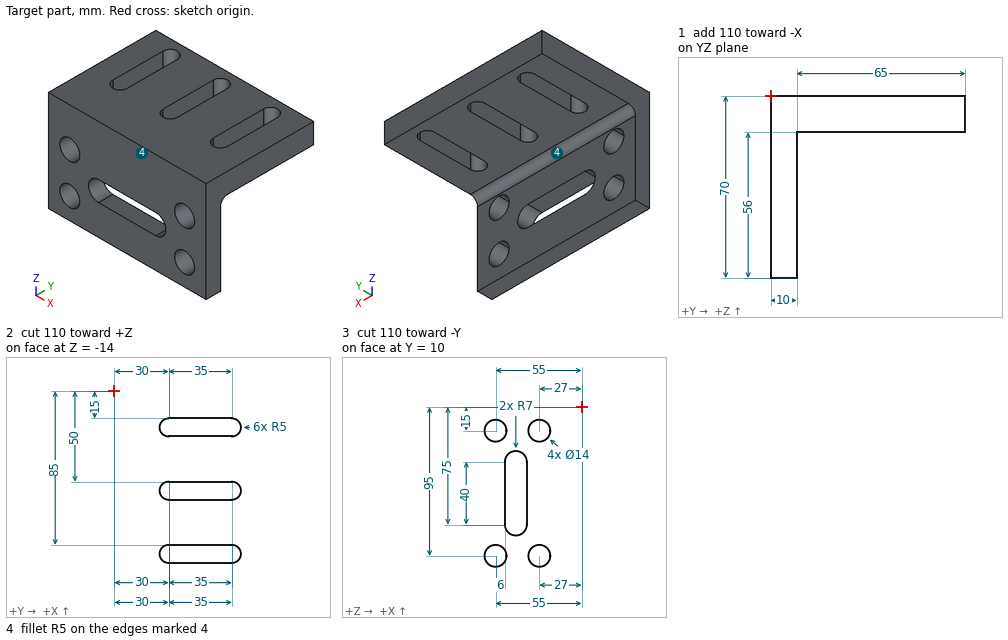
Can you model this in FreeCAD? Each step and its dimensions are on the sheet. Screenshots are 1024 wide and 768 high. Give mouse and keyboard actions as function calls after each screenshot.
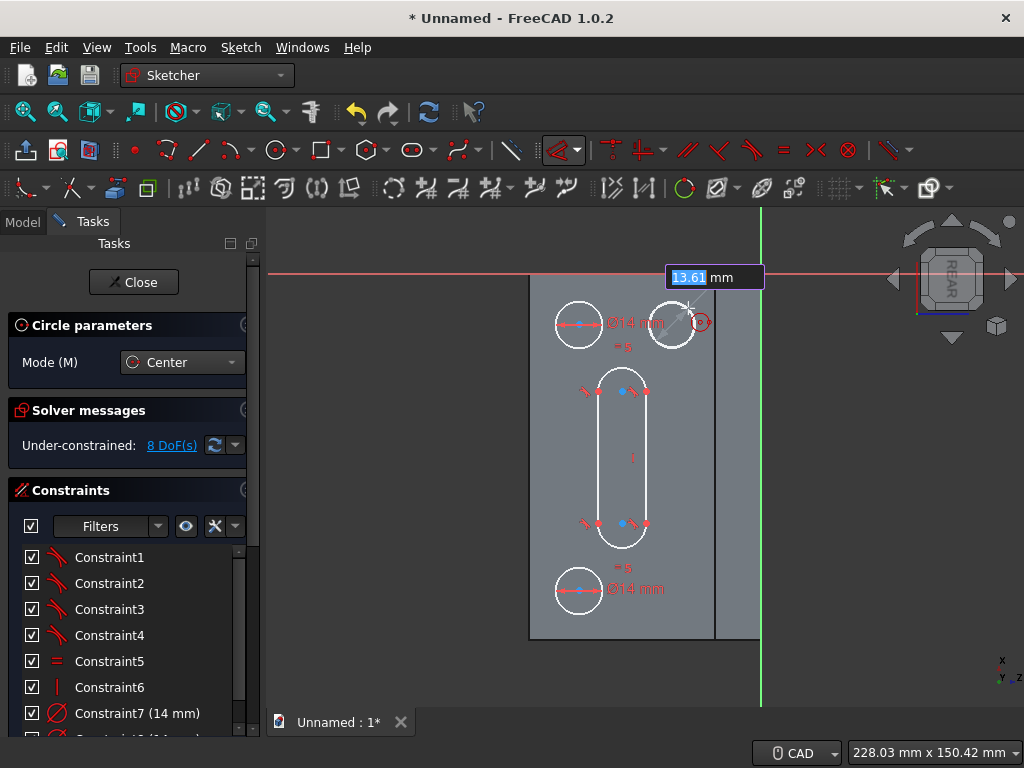
text(14)
key(Return)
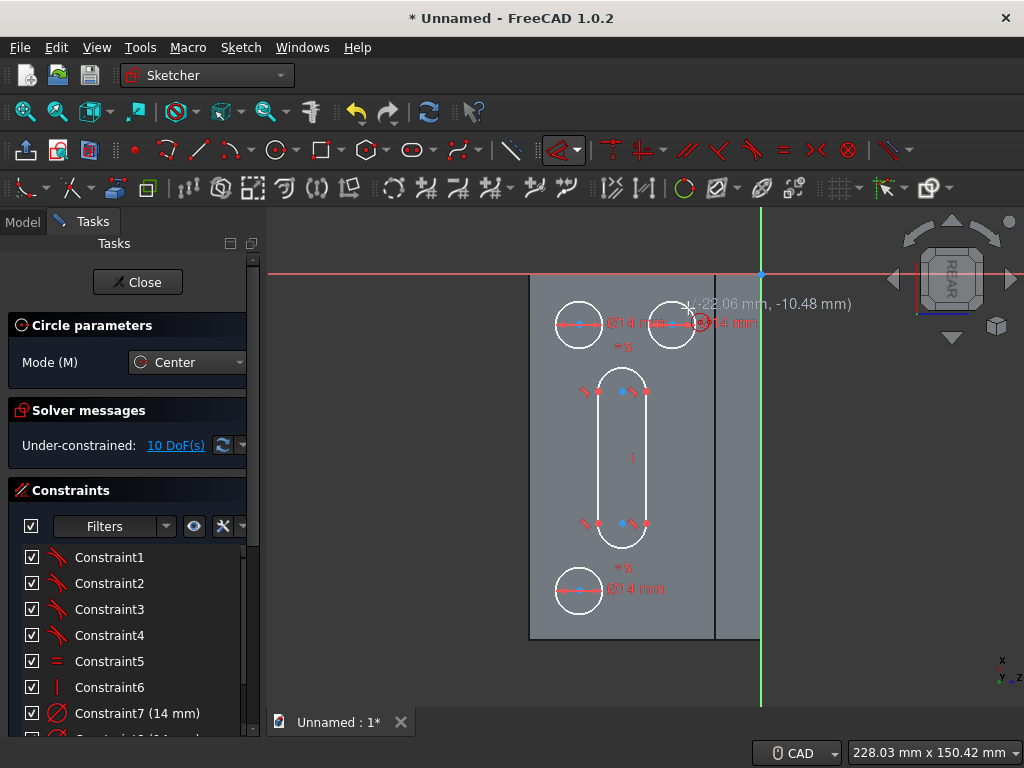
click(672, 590)
move(688, 574)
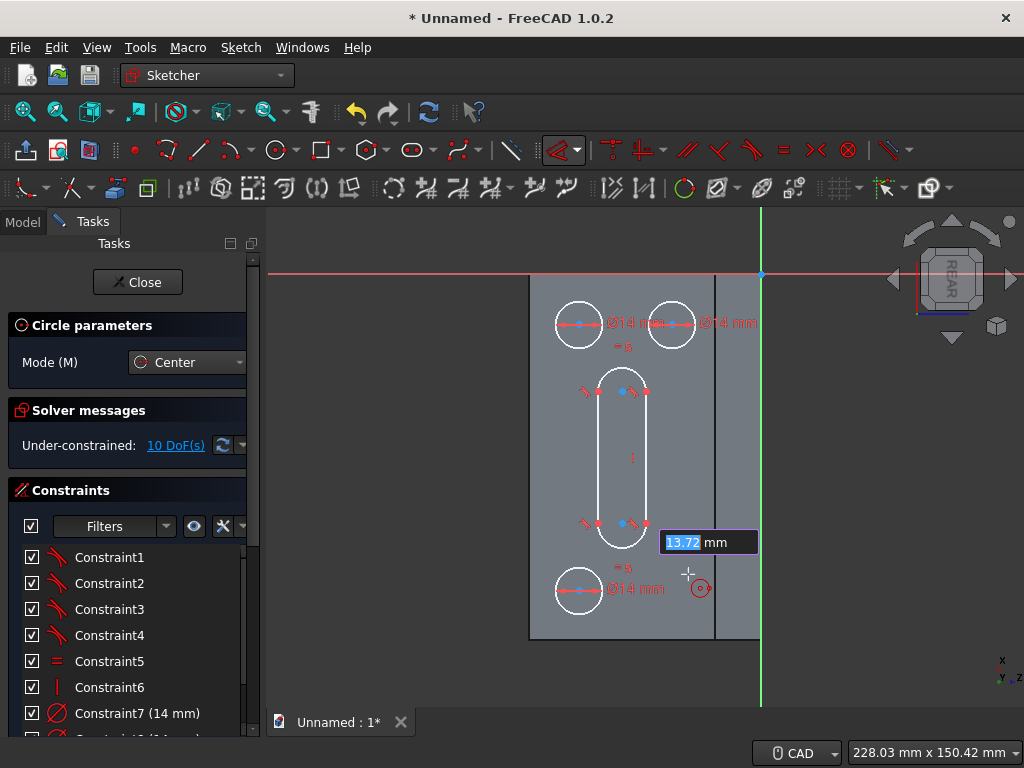
text(14)
key(Return)
key(Escape)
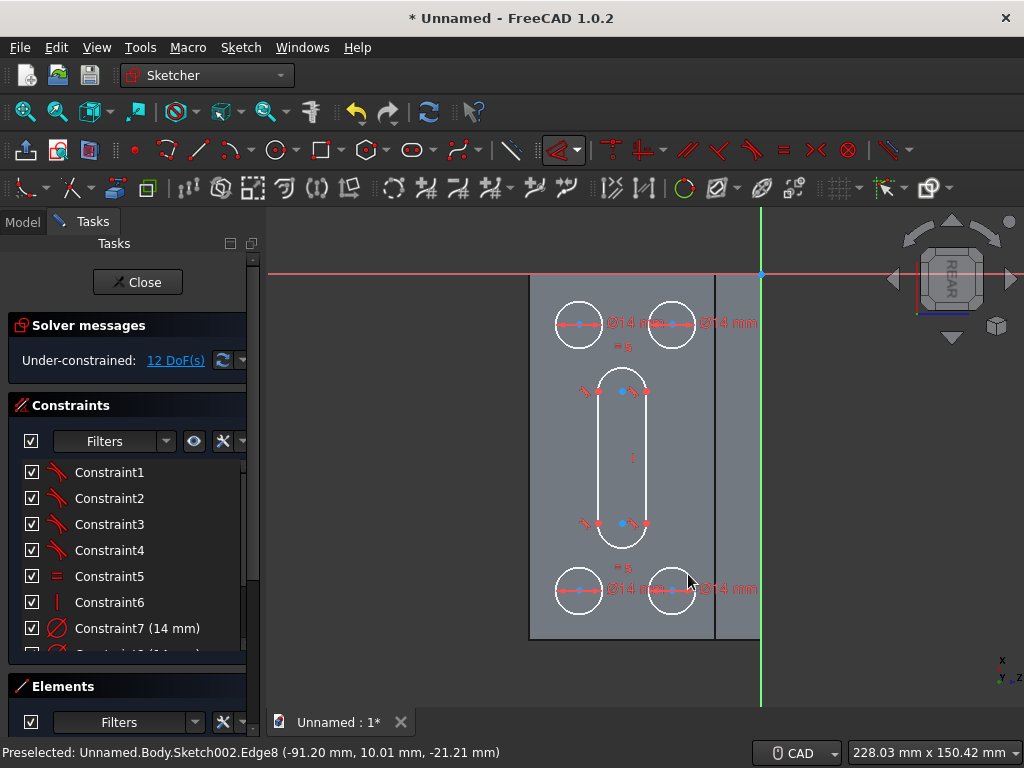
click(579, 325)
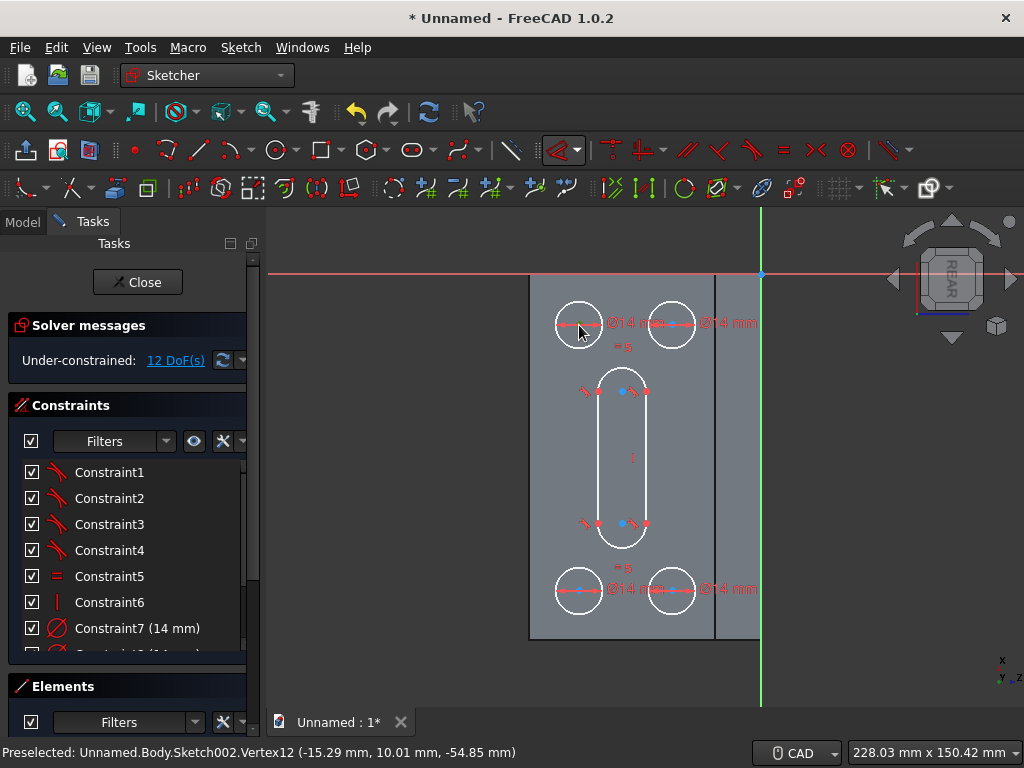
click(672, 325)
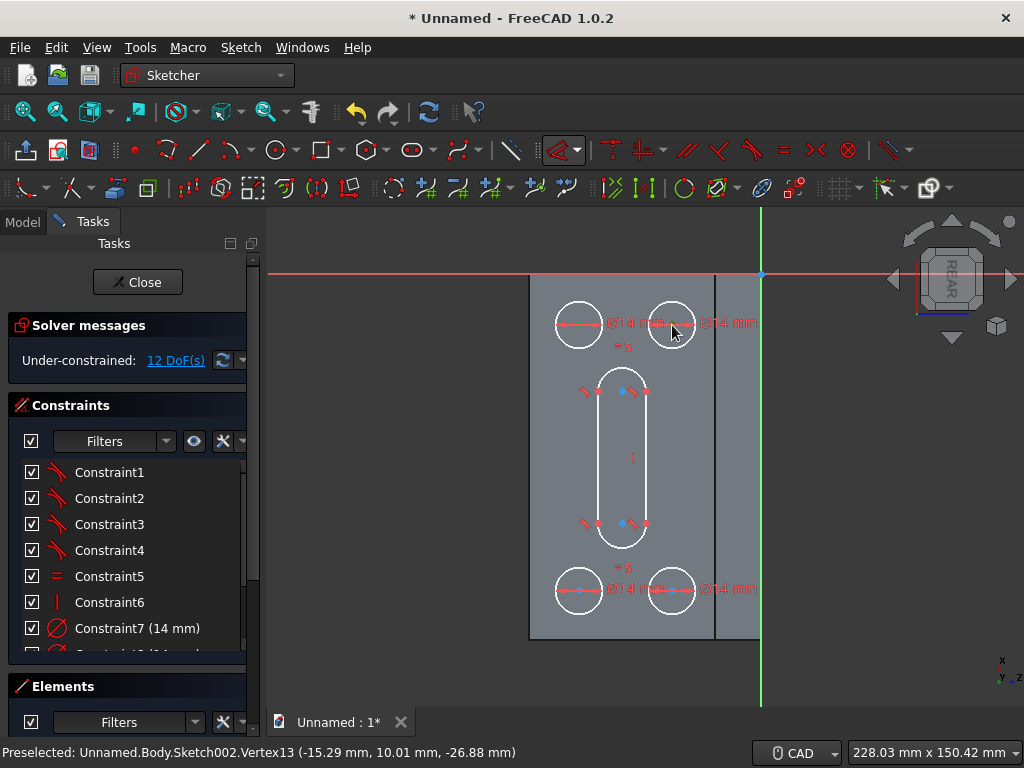
key(h)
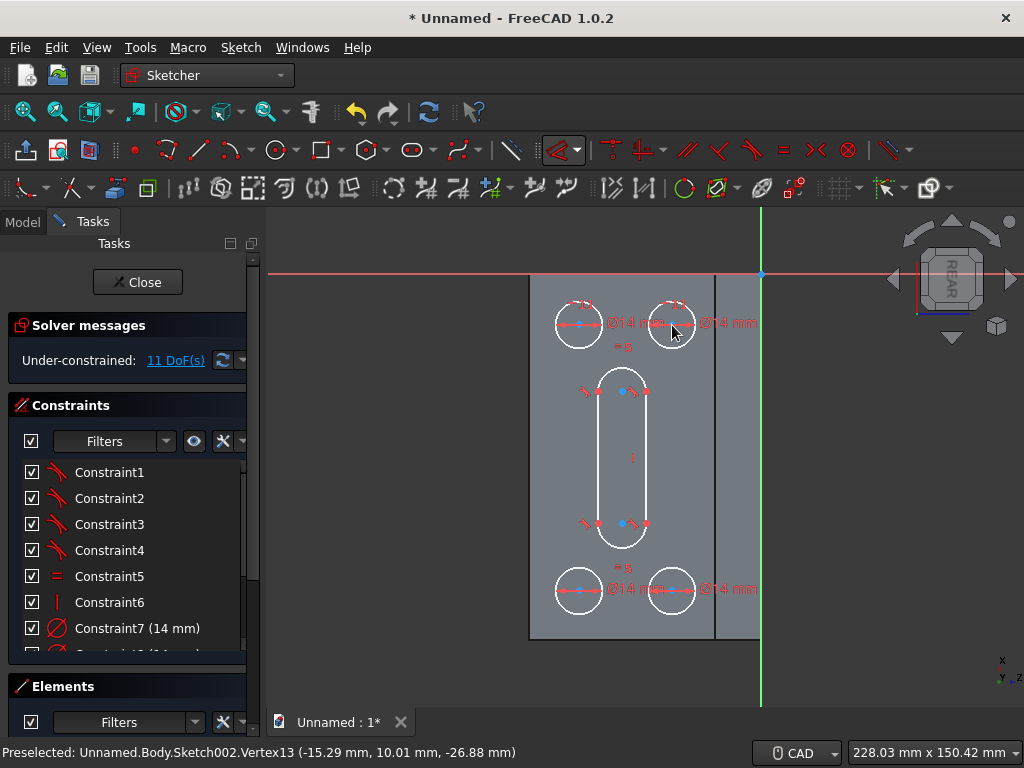
click(579, 591)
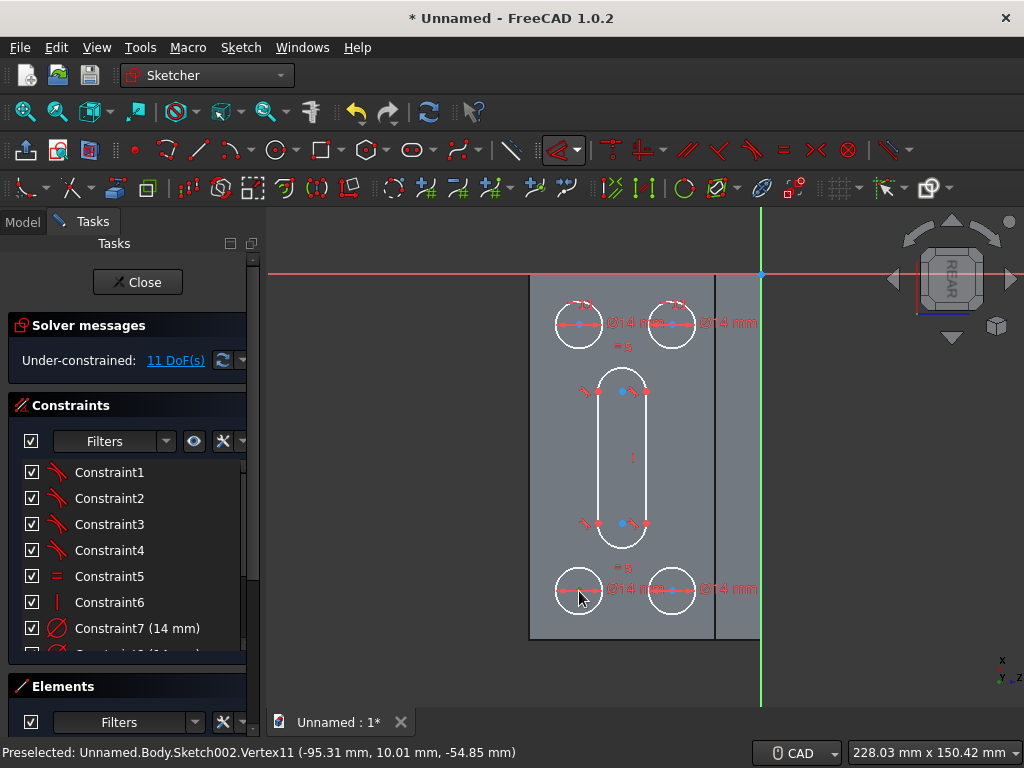
click(672, 591)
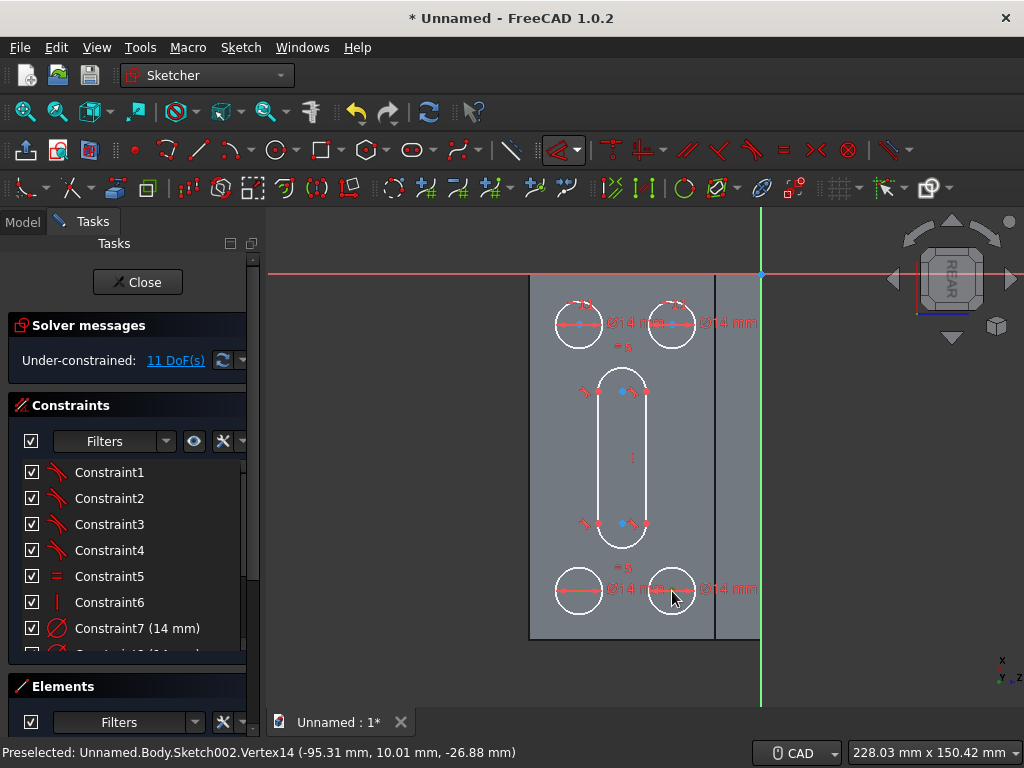
key(h)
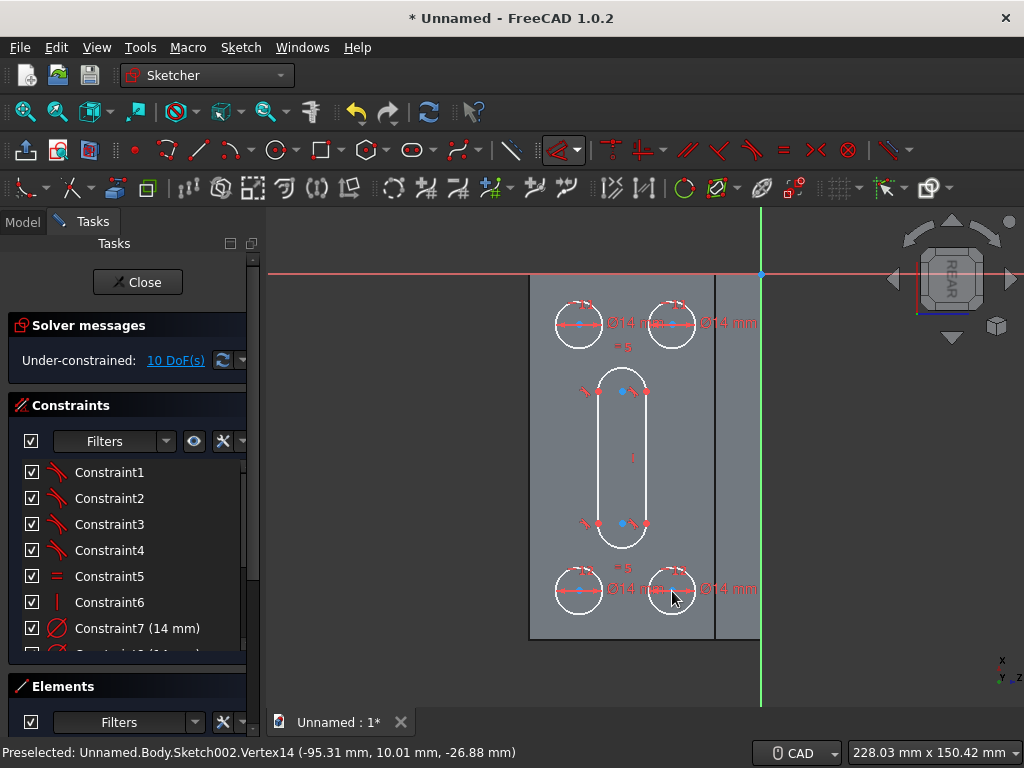
scroll(608, 543, up, 3)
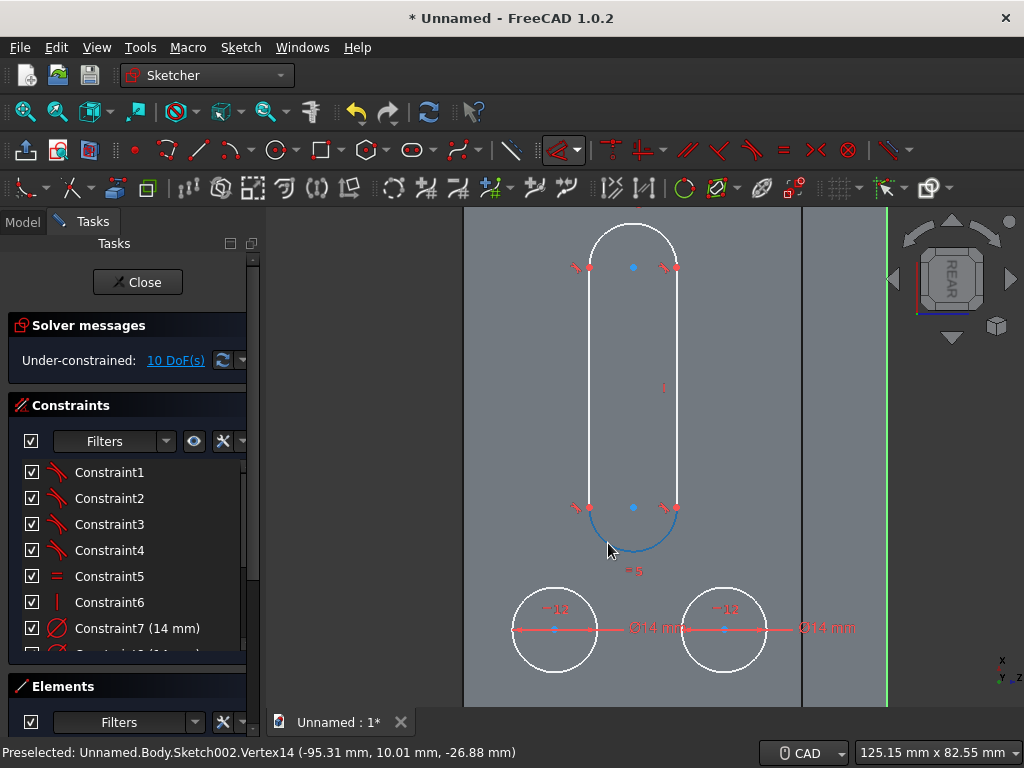
click(607, 543)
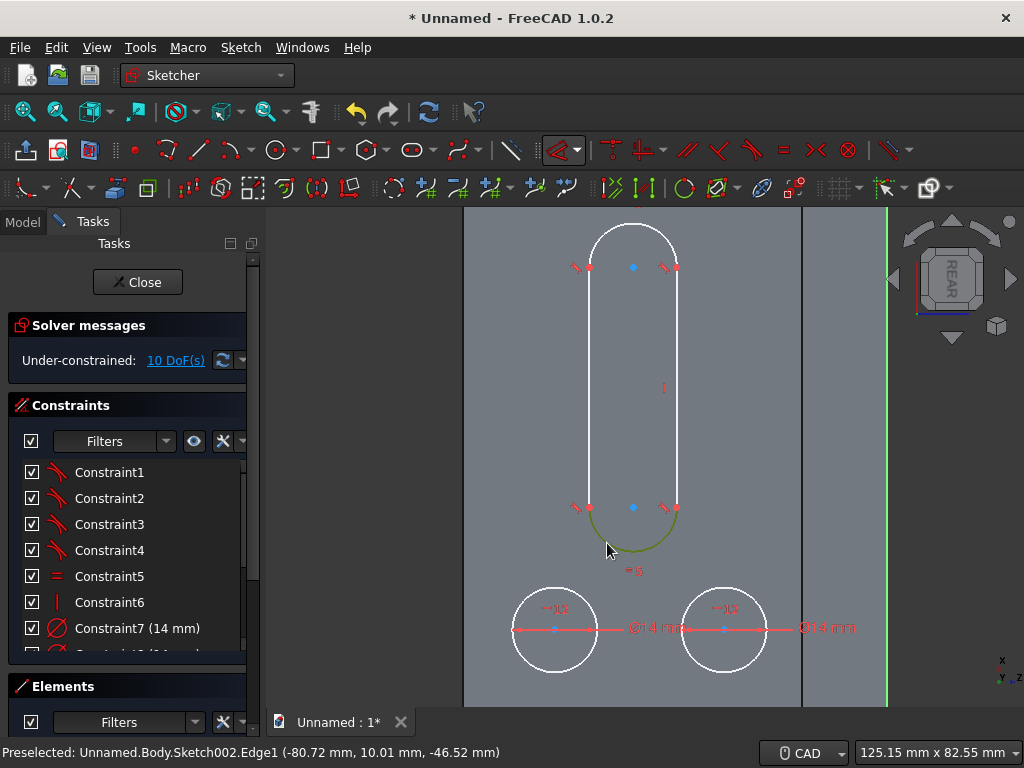
click(580, 150)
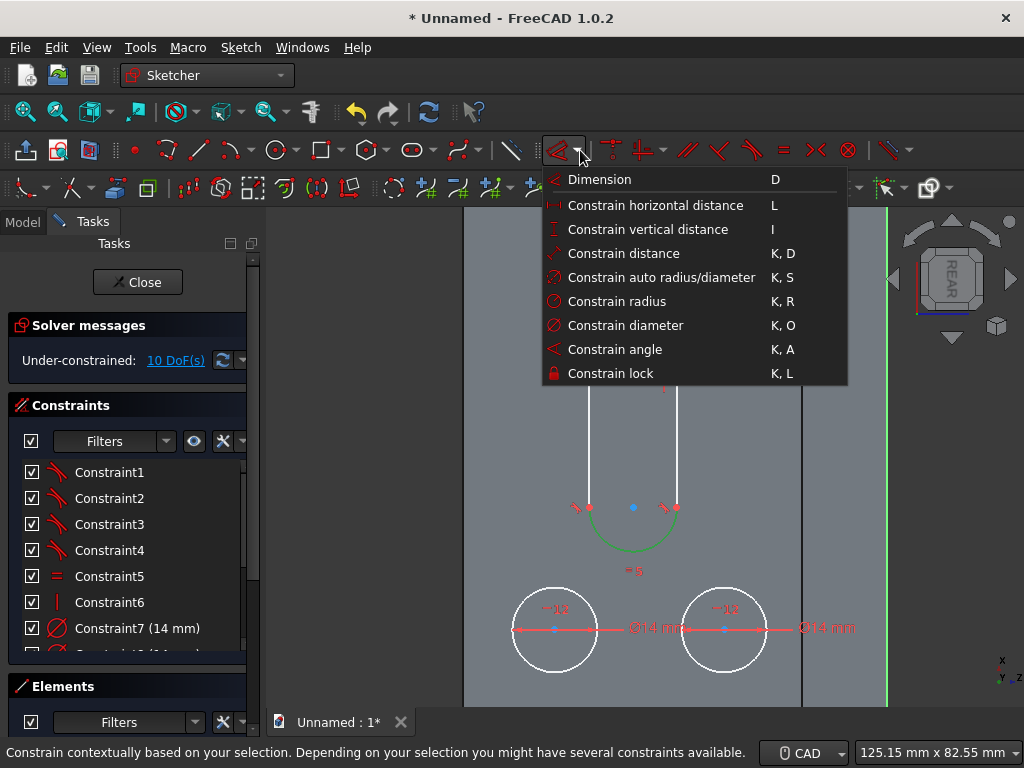
click(695, 301)